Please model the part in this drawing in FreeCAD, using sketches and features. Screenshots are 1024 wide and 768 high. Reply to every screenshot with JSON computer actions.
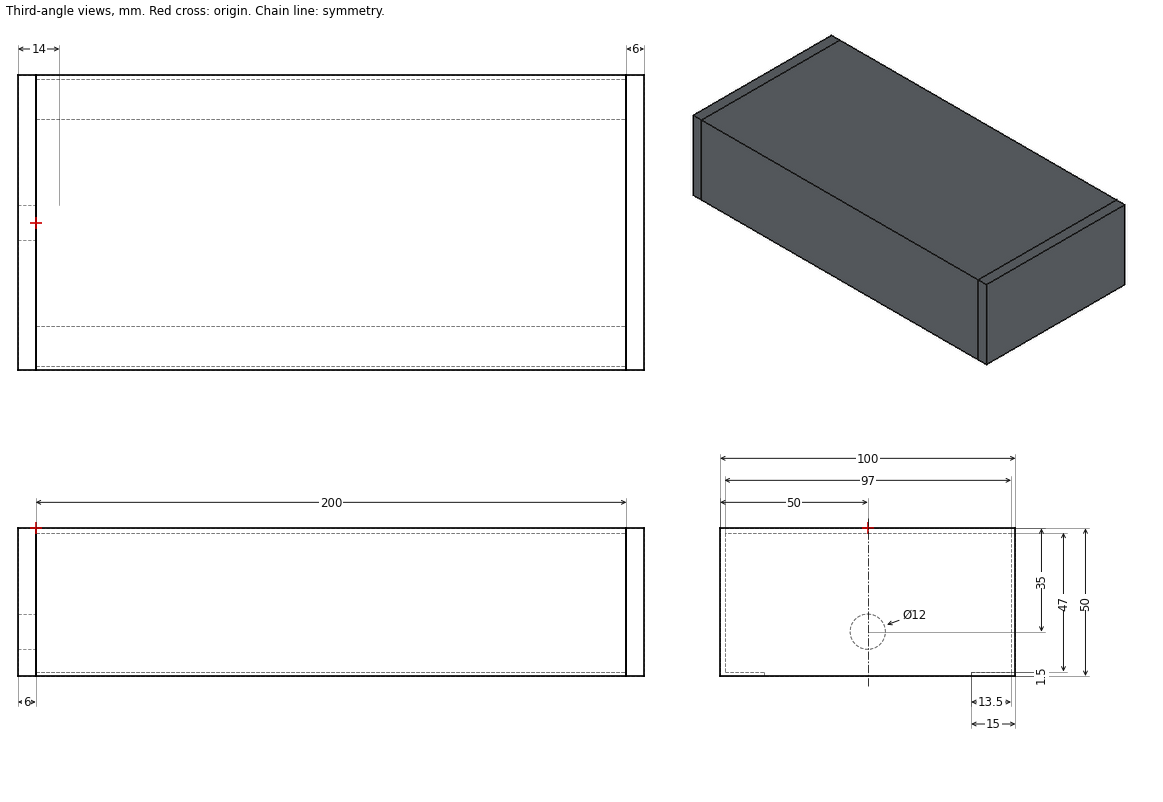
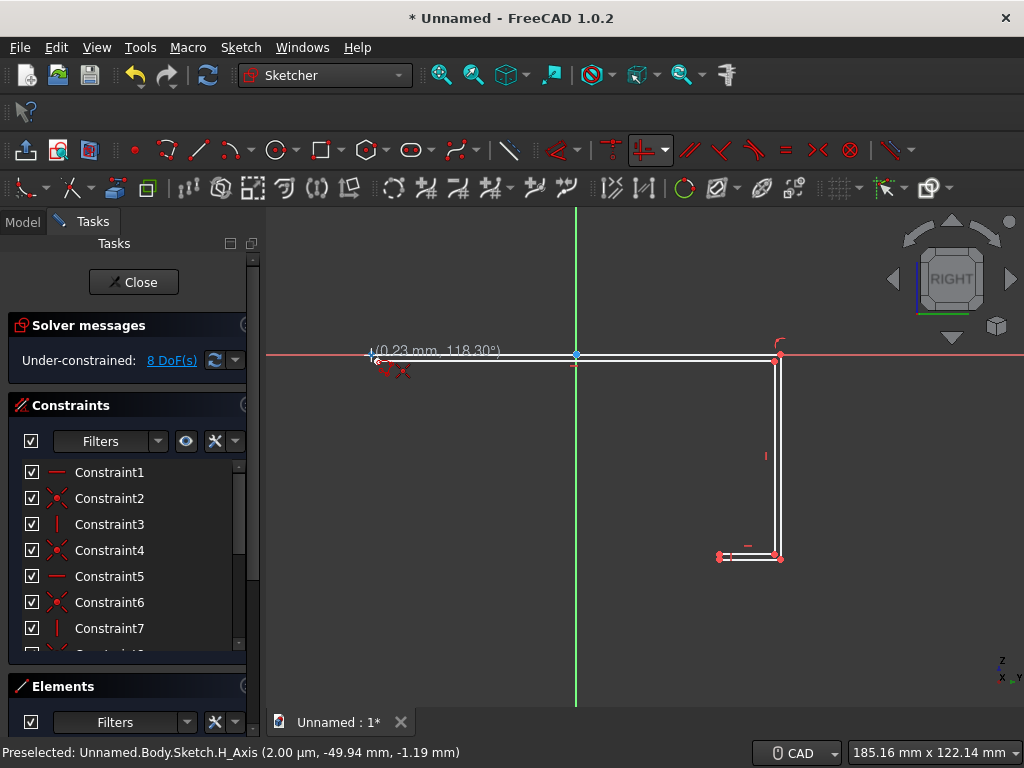
{"action": "left_click", "coordinate": [372, 559]}
{"action": "left_click", "coordinate": [433, 559]}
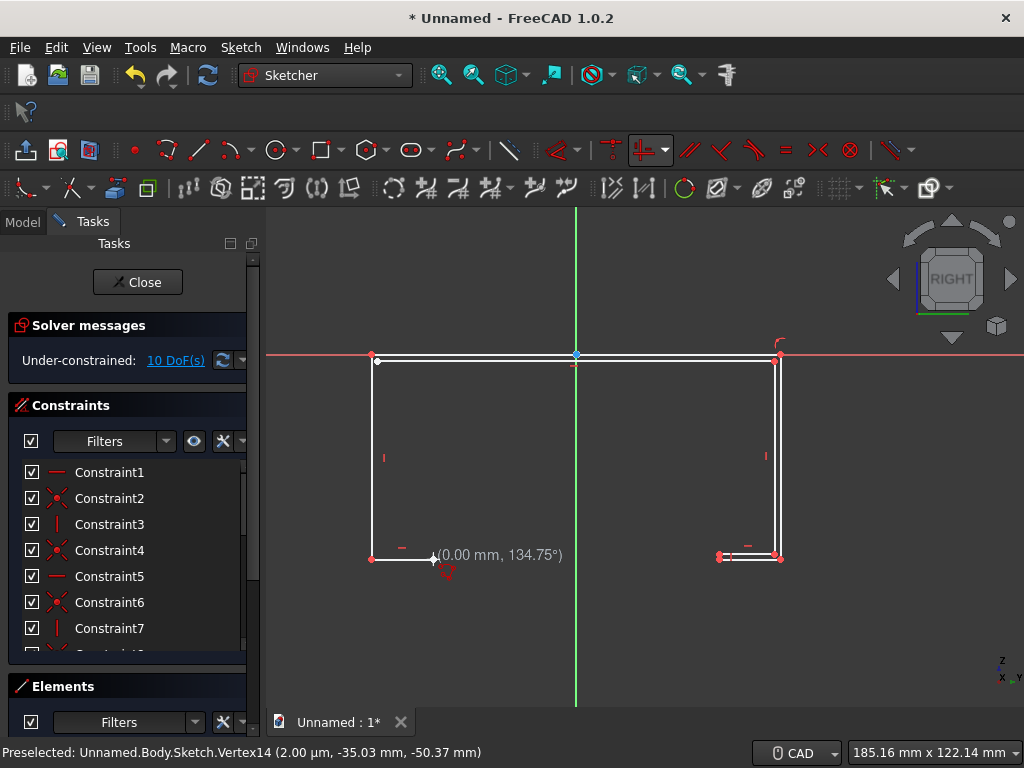
{"action": "scroll", "coordinate": [433, 553], "scroll_direction": "up", "scroll_amount": 5}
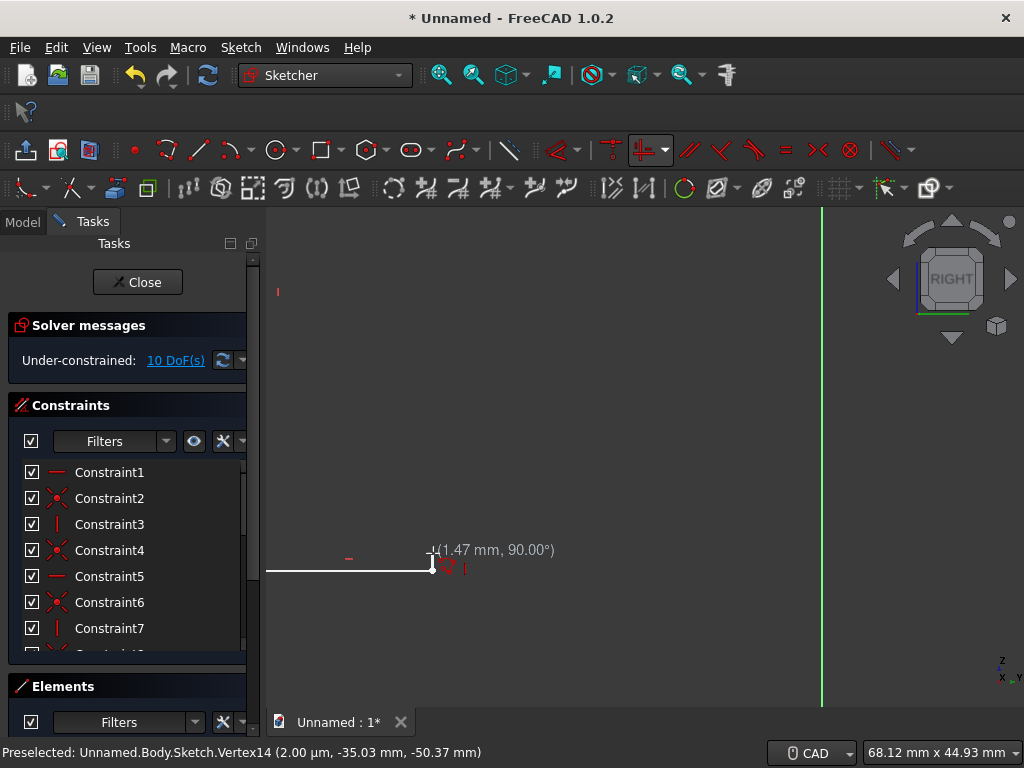
{"action": "left_click", "coordinate": [433, 553]}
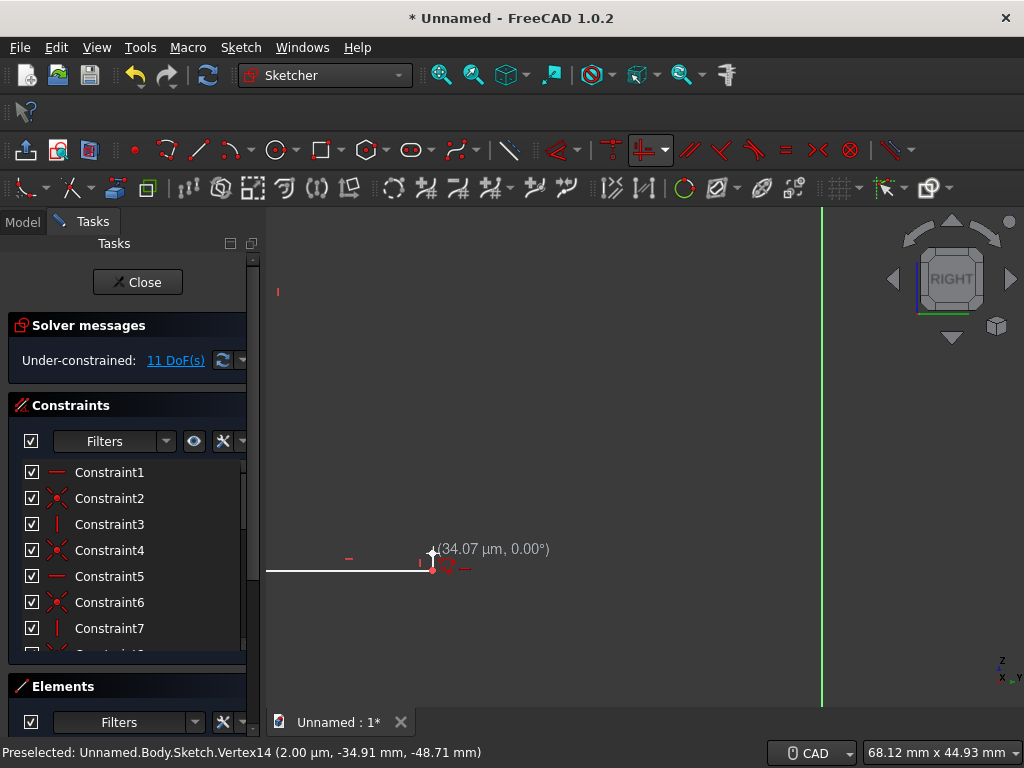
{"action": "scroll", "coordinate": [433, 554], "scroll_direction": "down", "scroll_amount": 5}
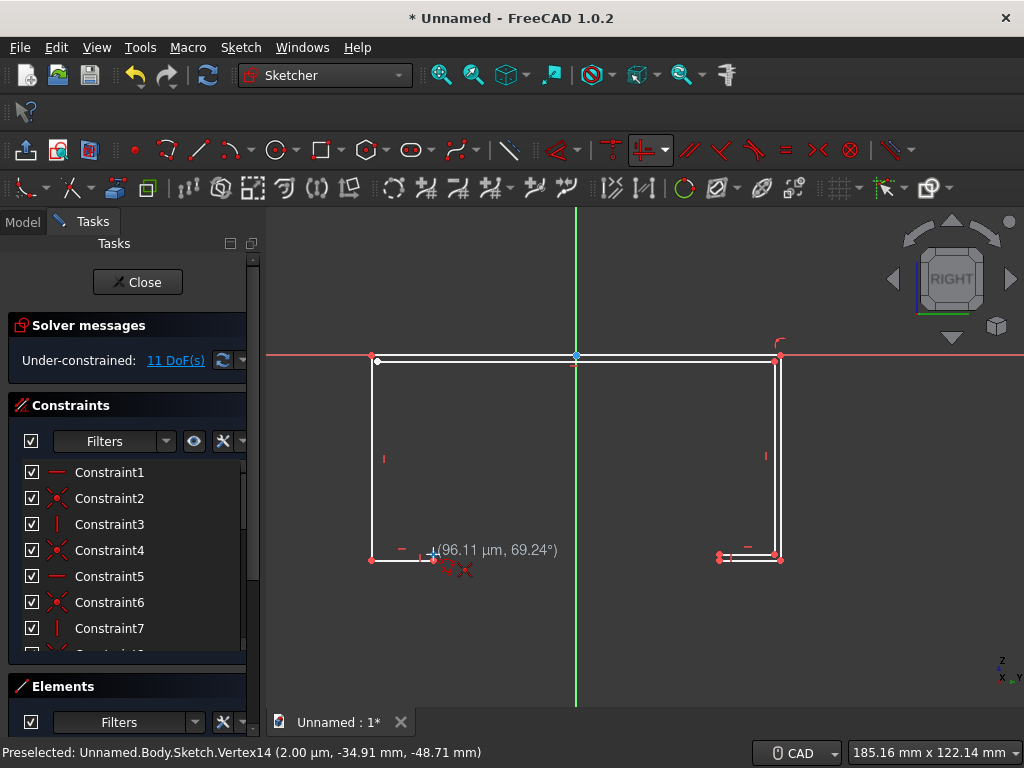
{"action": "scroll", "coordinate": [378, 554], "scroll_direction": "up", "scroll_amount": 5}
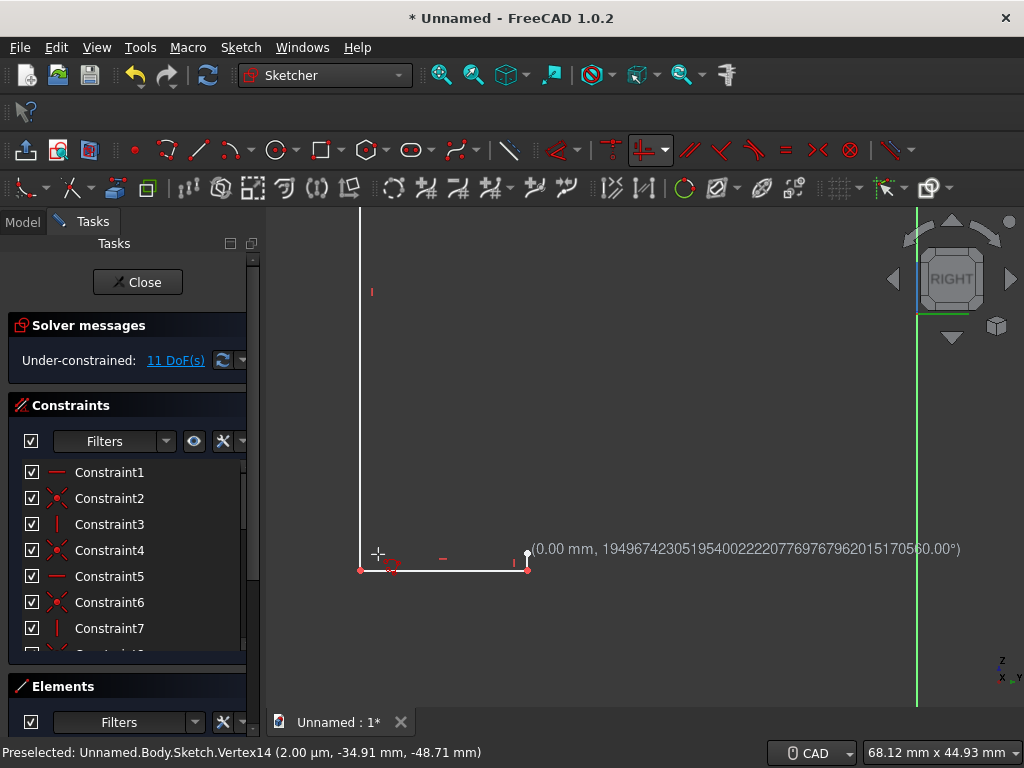
{"action": "left_click", "coordinate": [377, 553]}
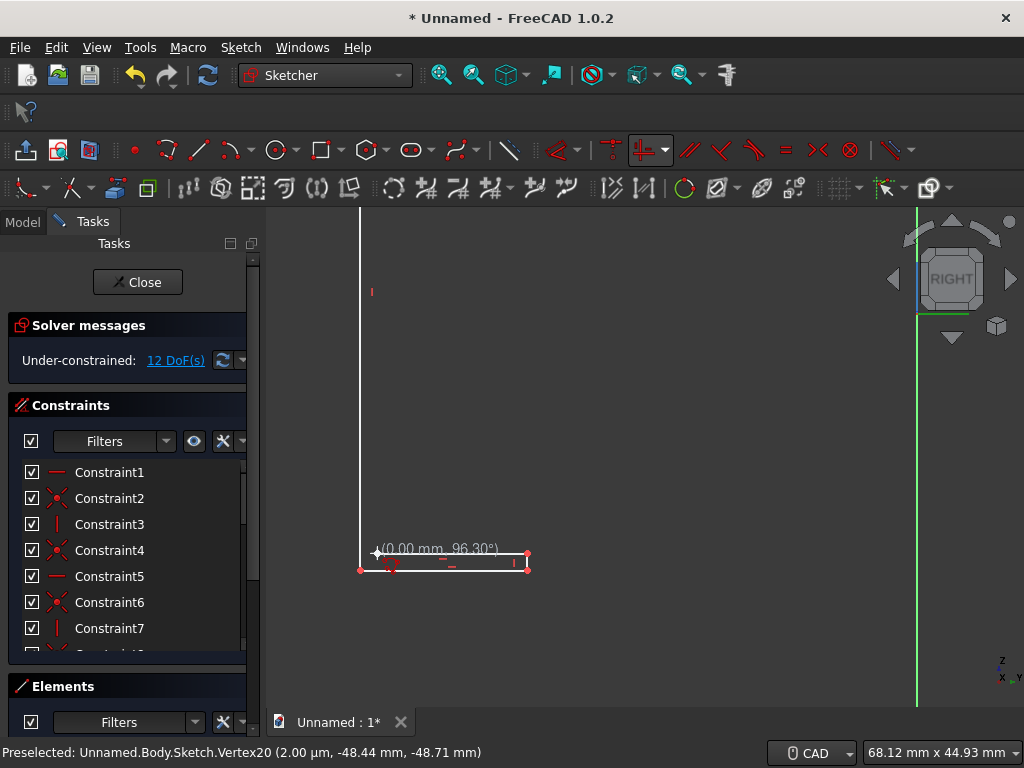
{"action": "scroll", "coordinate": [378, 554], "scroll_direction": "down", "scroll_amount": 5}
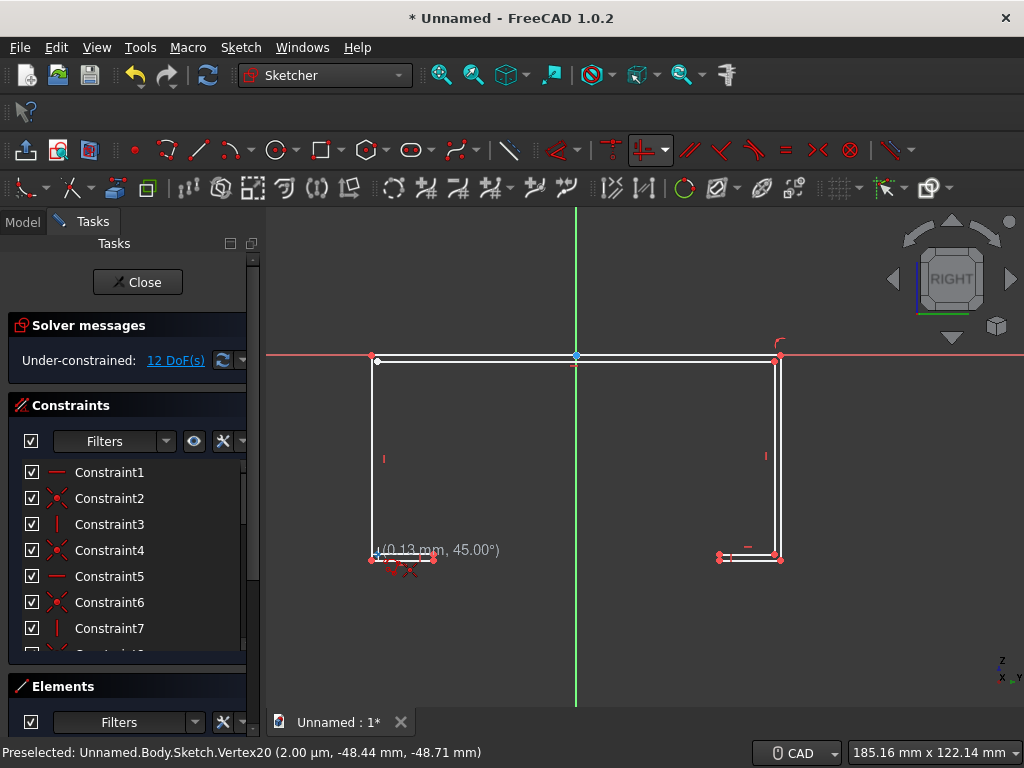
{"action": "scroll", "coordinate": [378, 362], "scroll_direction": "up", "scroll_amount": 5}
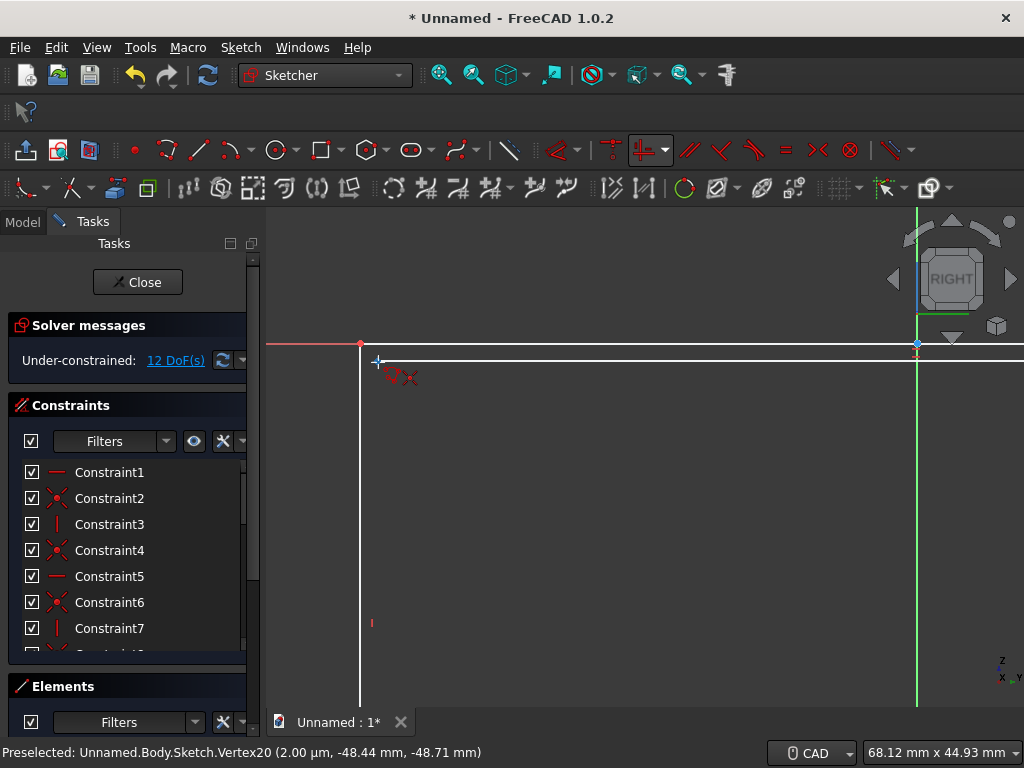
{"action": "left_click", "coordinate": [377, 361]}
{"action": "key", "text": "Escape"}
{"action": "key", "text": "Escape"}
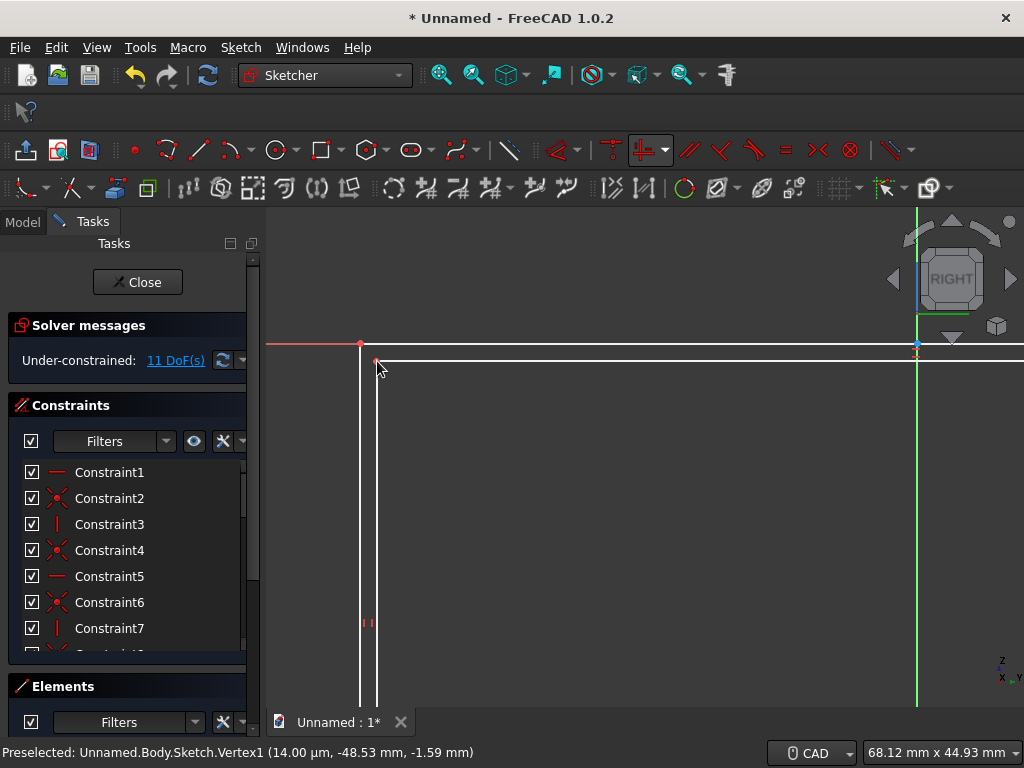
{"action": "scroll", "coordinate": [378, 361], "scroll_direction": "down", "scroll_amount": 5}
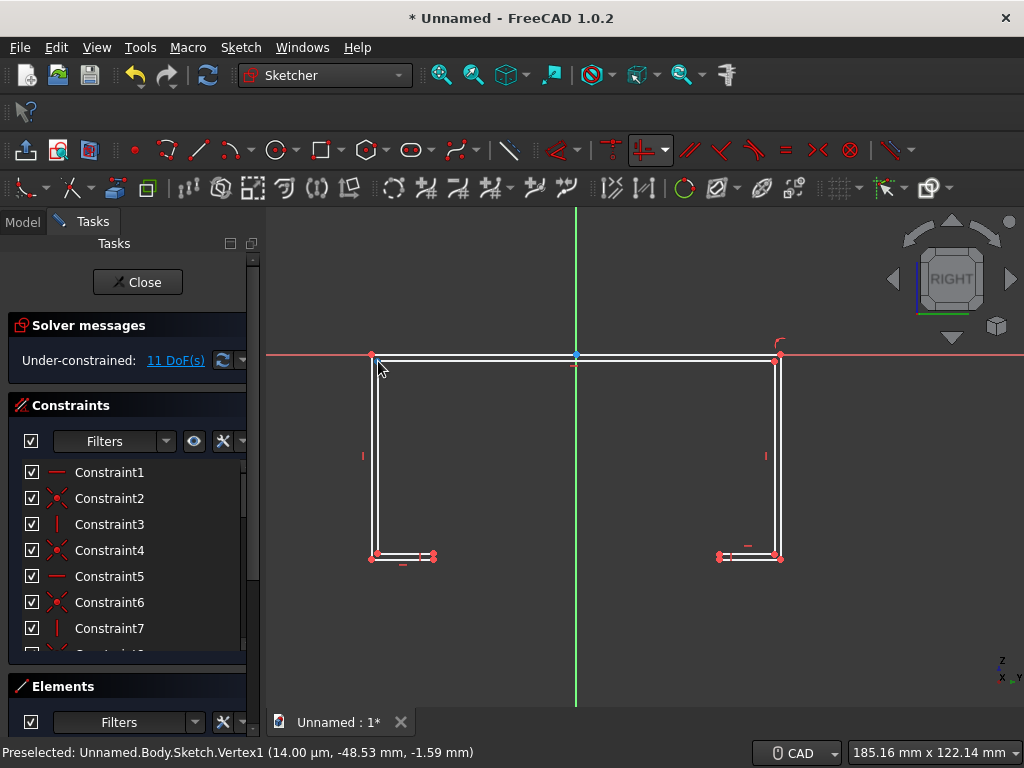
{"action": "scroll", "coordinate": [781, 560], "scroll_direction": "up", "scroll_amount": 2}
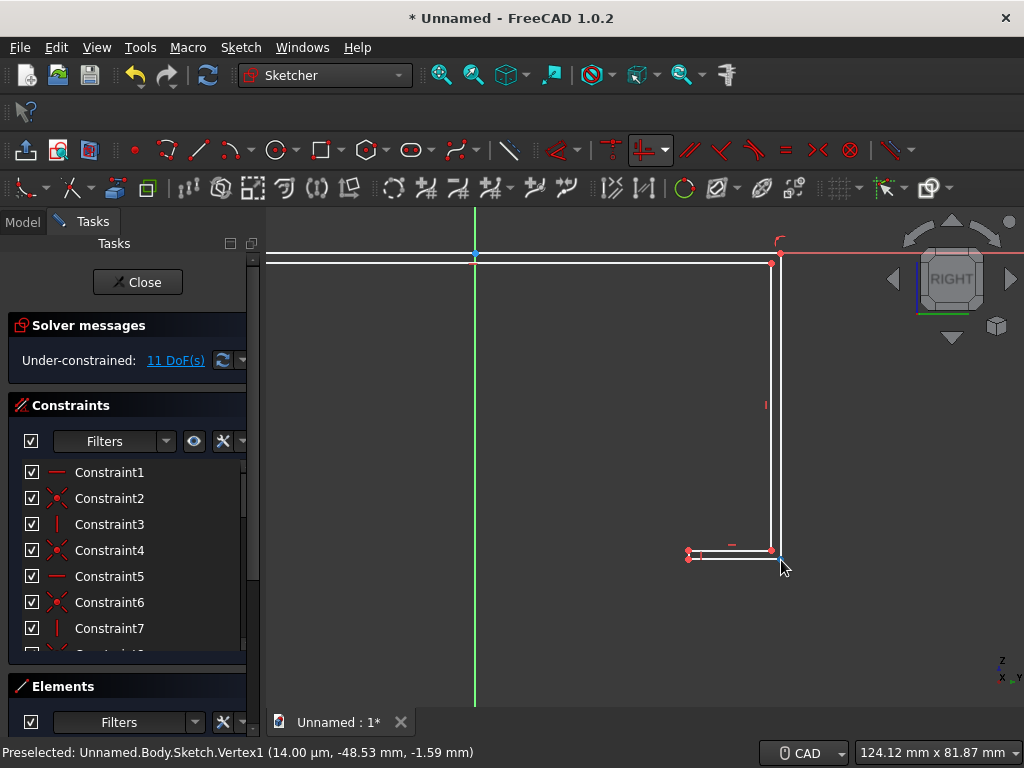
{"action": "left_click", "coordinate": [781, 559]}